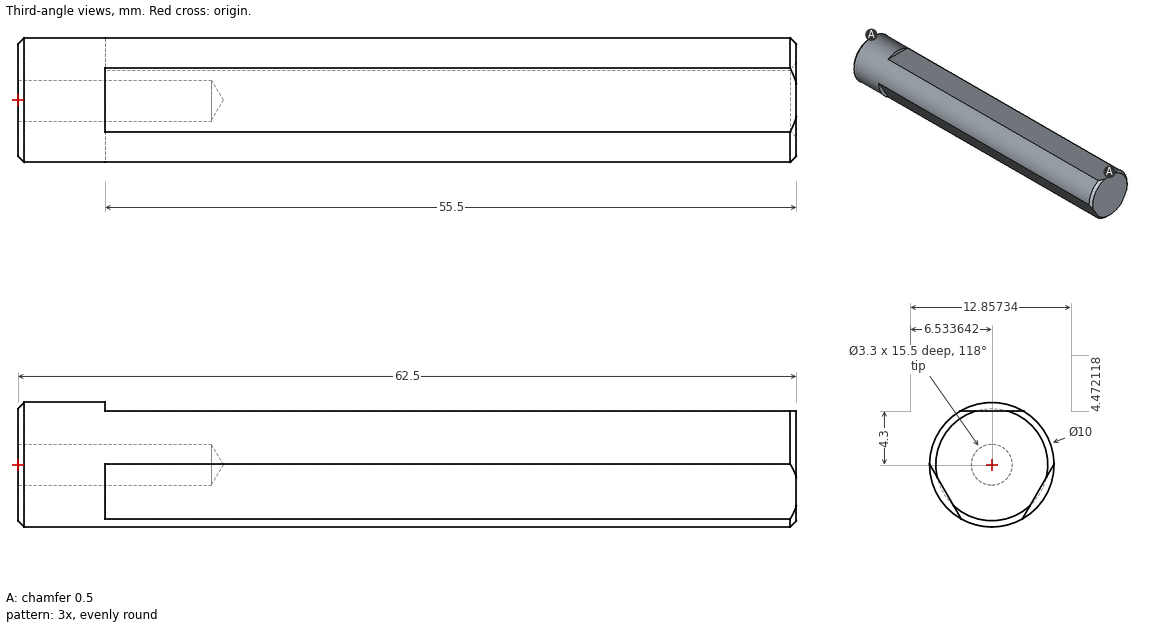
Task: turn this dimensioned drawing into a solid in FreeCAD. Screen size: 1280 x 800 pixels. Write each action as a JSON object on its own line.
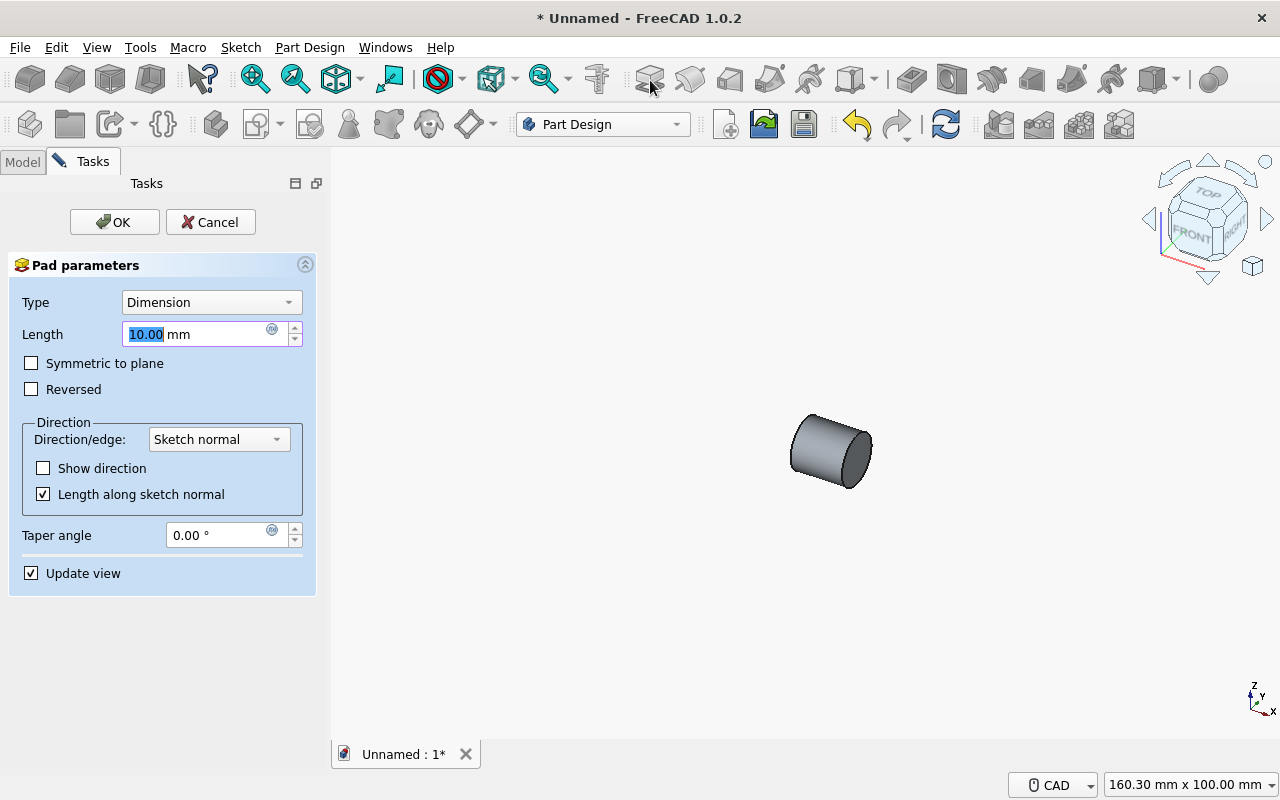
{"action": "type", "text": "62.5"}
{"action": "key", "text": "Tab"}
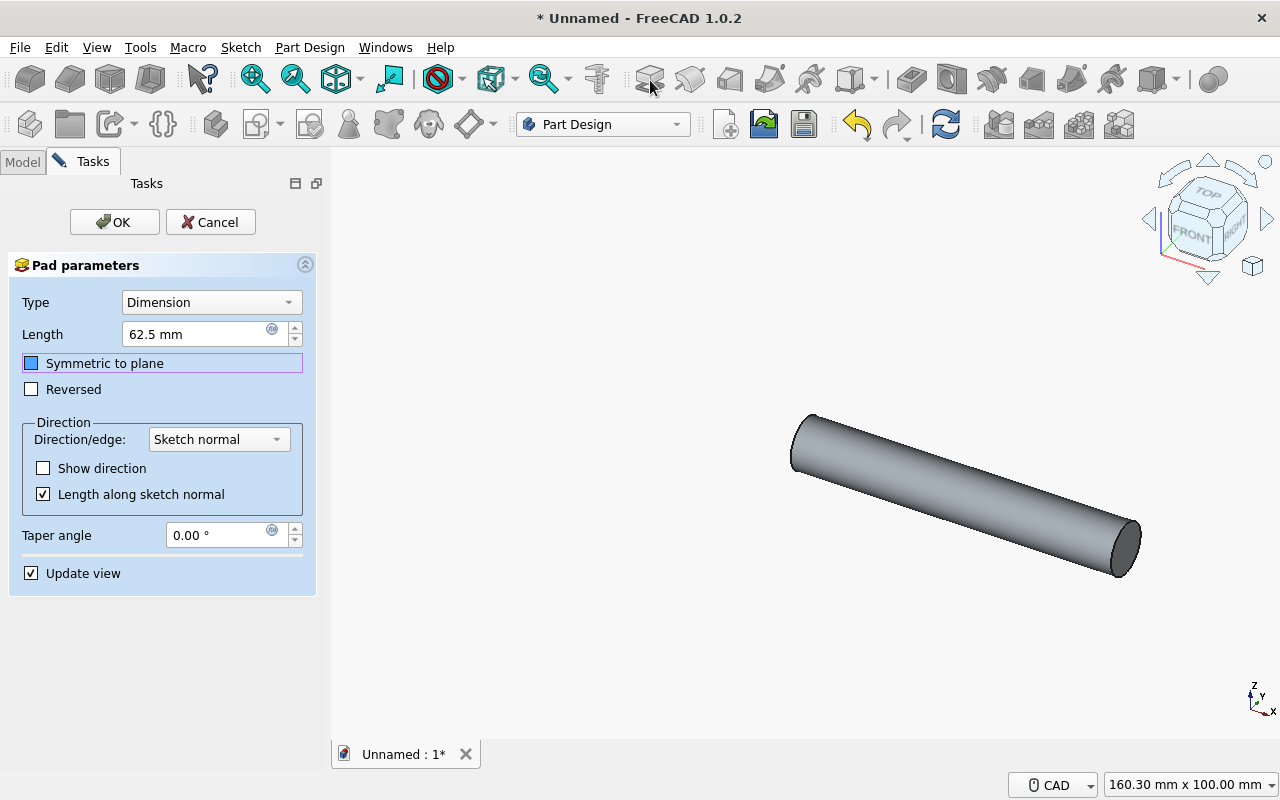
{"action": "left_click", "coordinate": [115, 222]}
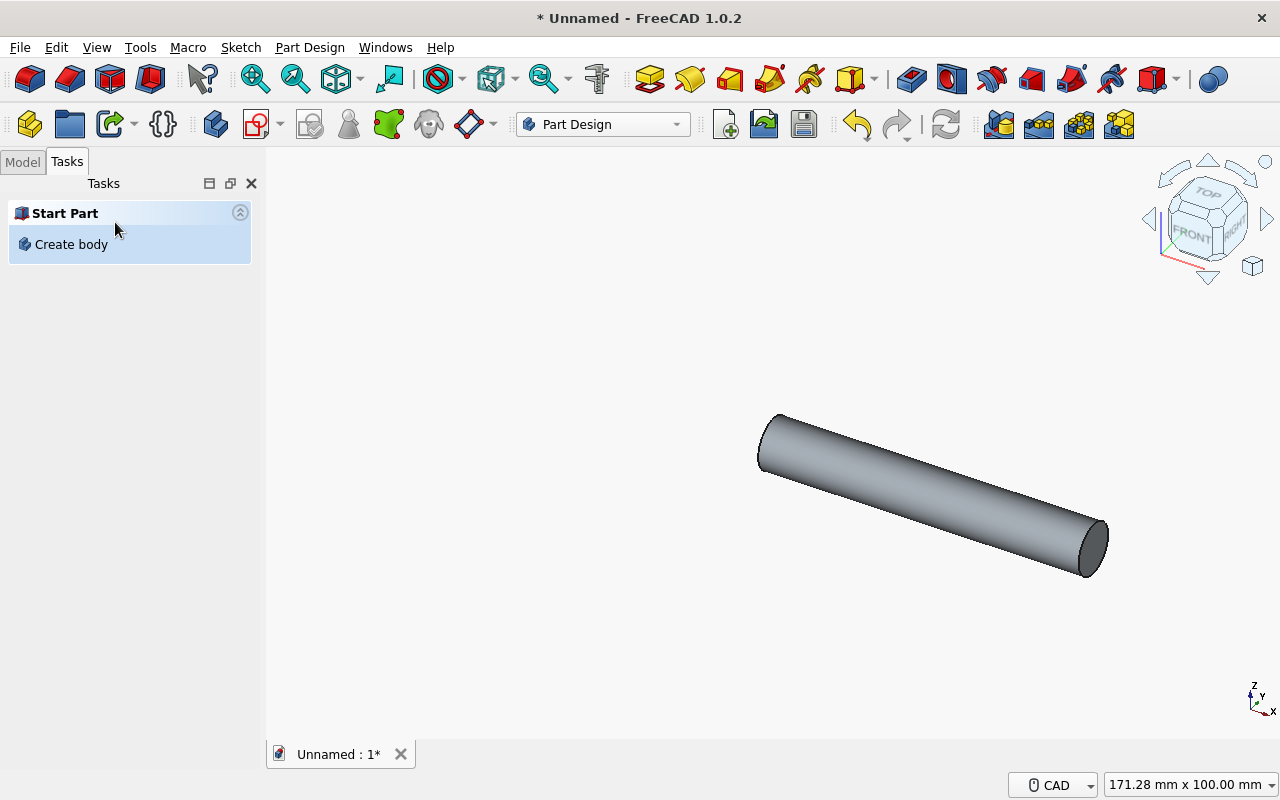
{"action": "left_click", "coordinate": [256, 80]}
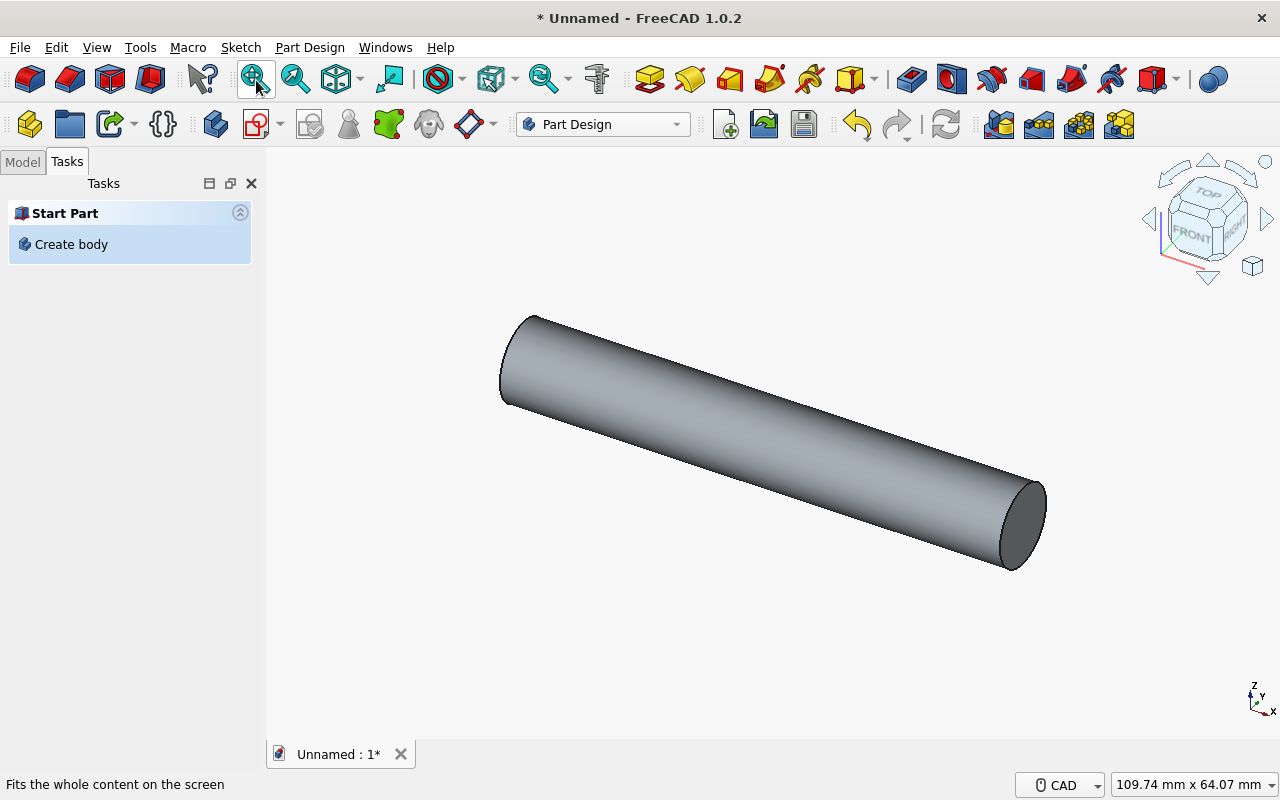
{"action": "left_click", "coordinate": [1000, 548]}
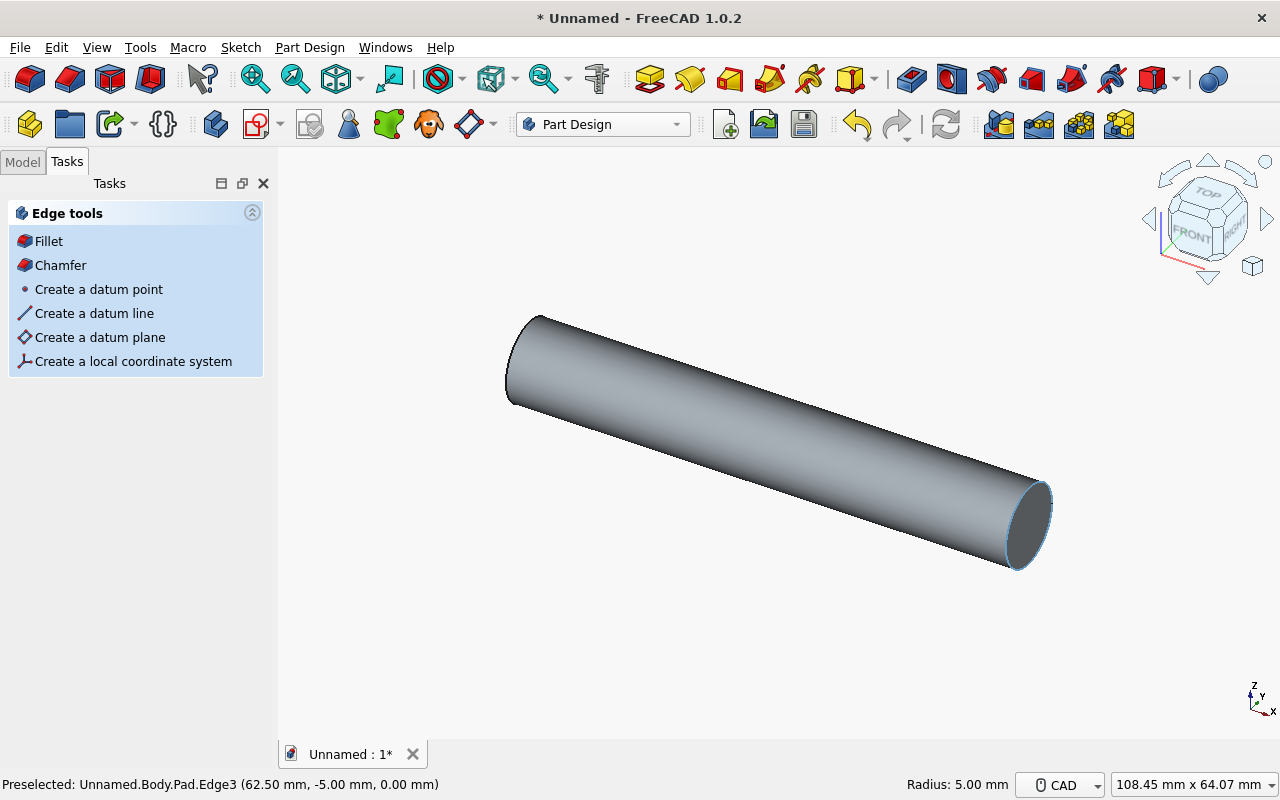
{"action": "key", "text": "0"}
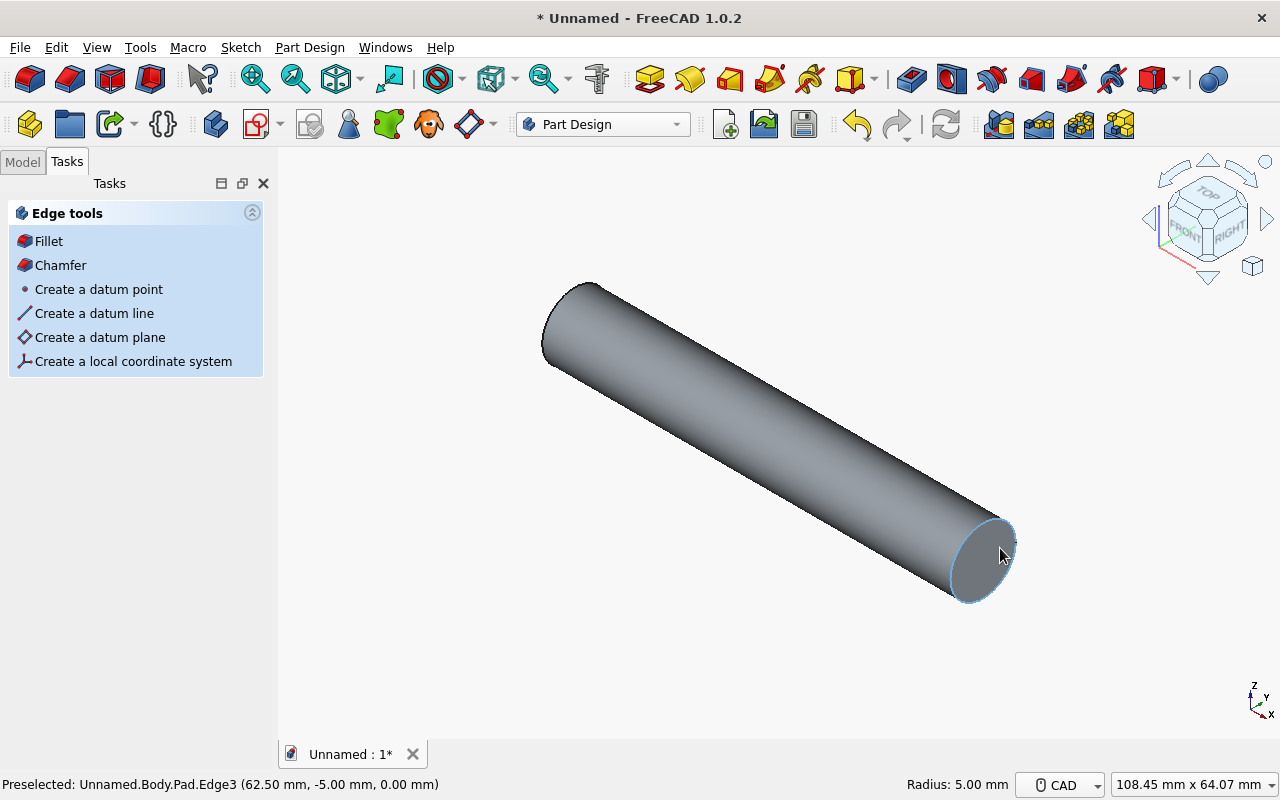
{"action": "key", "text": "2"}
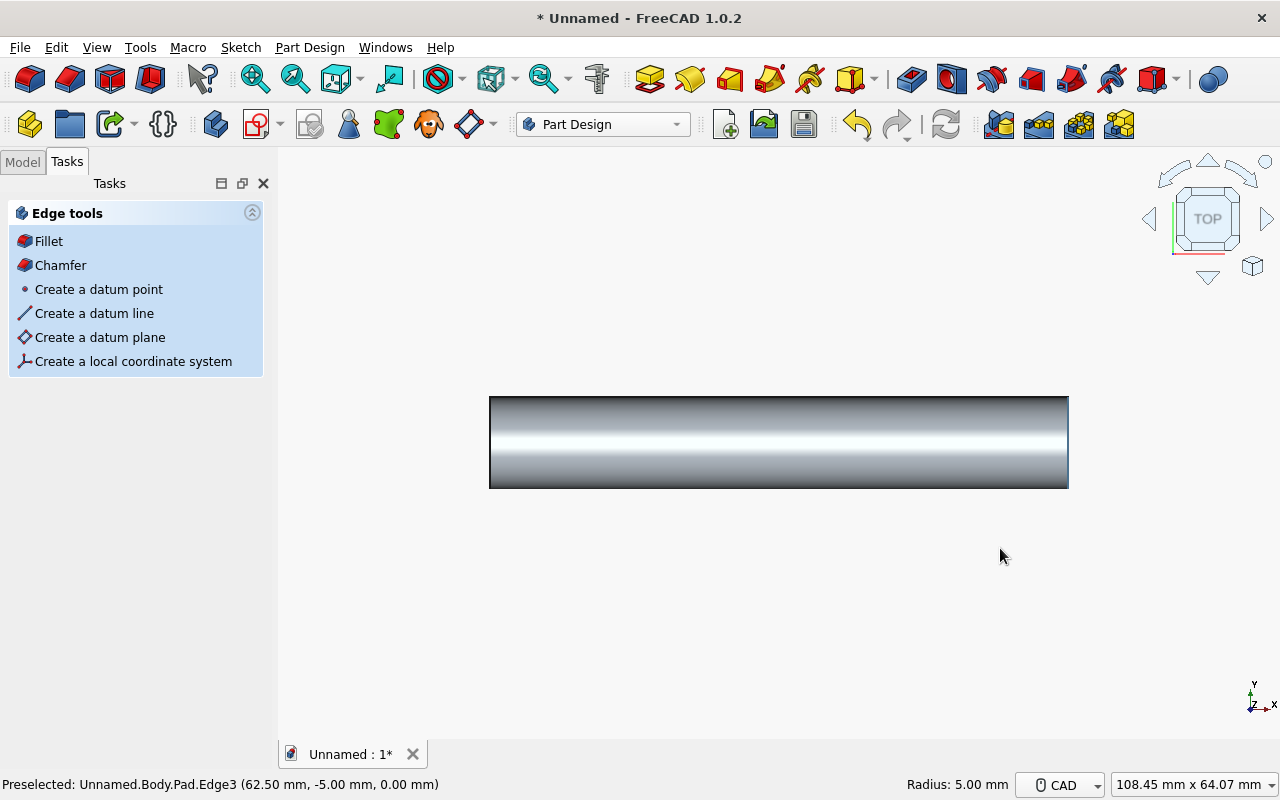
{"action": "left_click", "coordinate": [490, 479], "text": "ctrl"}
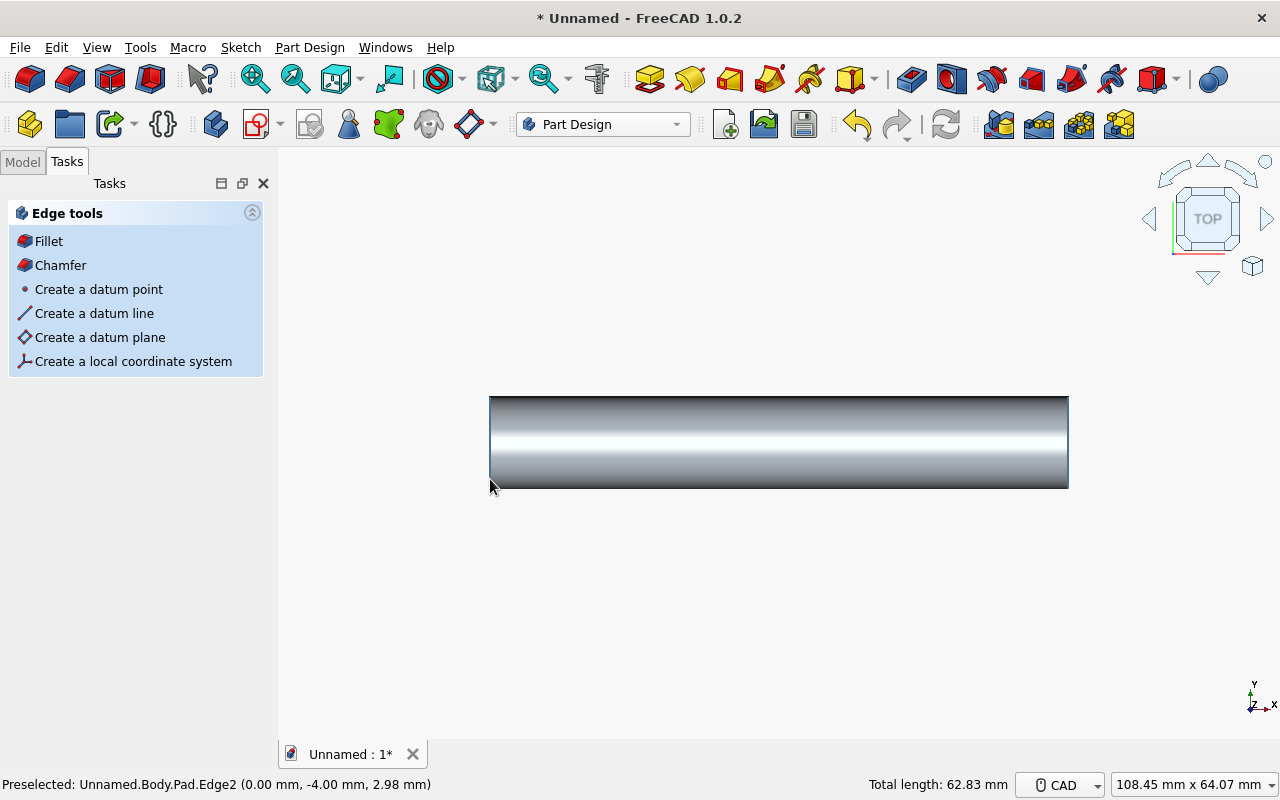
{"action": "left_click", "coordinate": [70, 80]}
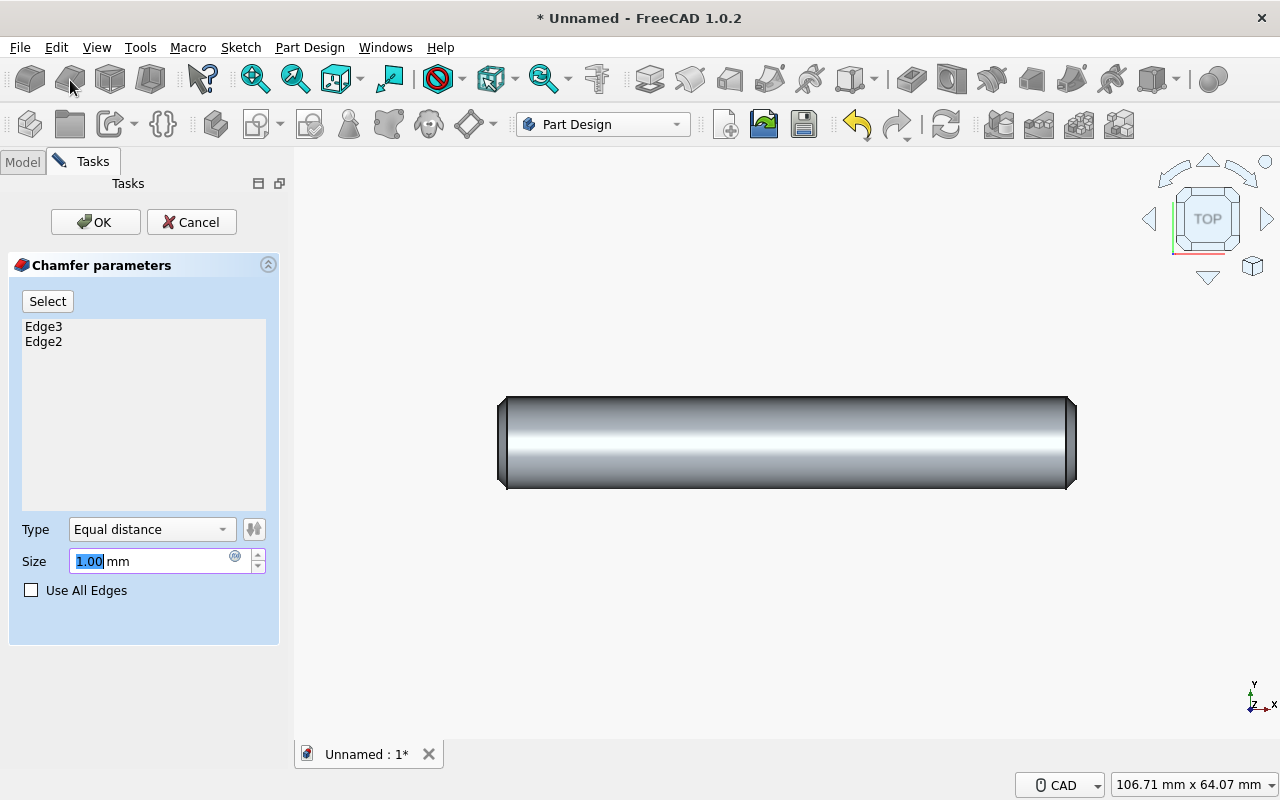
{"action": "type", "text": "0.5"}
{"action": "key", "text": "Tab"}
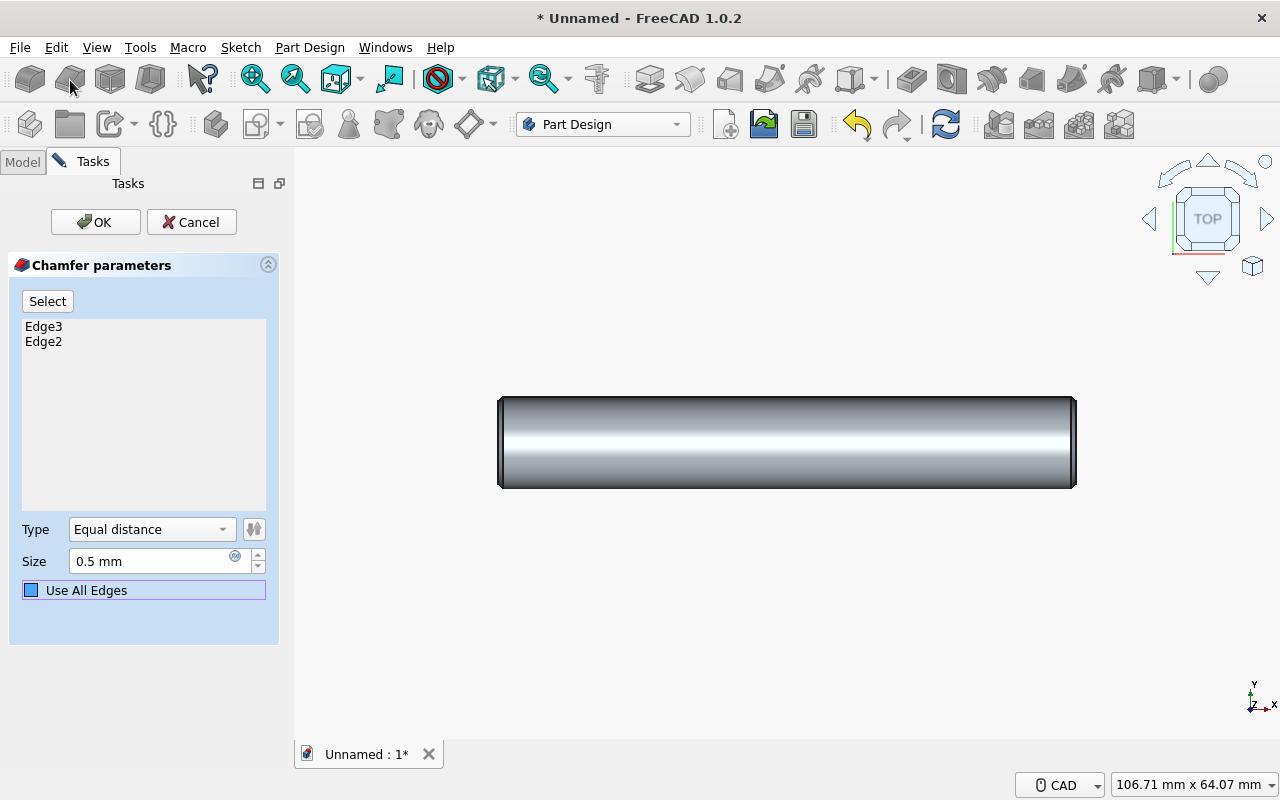
{"action": "left_click", "coordinate": [96, 222]}